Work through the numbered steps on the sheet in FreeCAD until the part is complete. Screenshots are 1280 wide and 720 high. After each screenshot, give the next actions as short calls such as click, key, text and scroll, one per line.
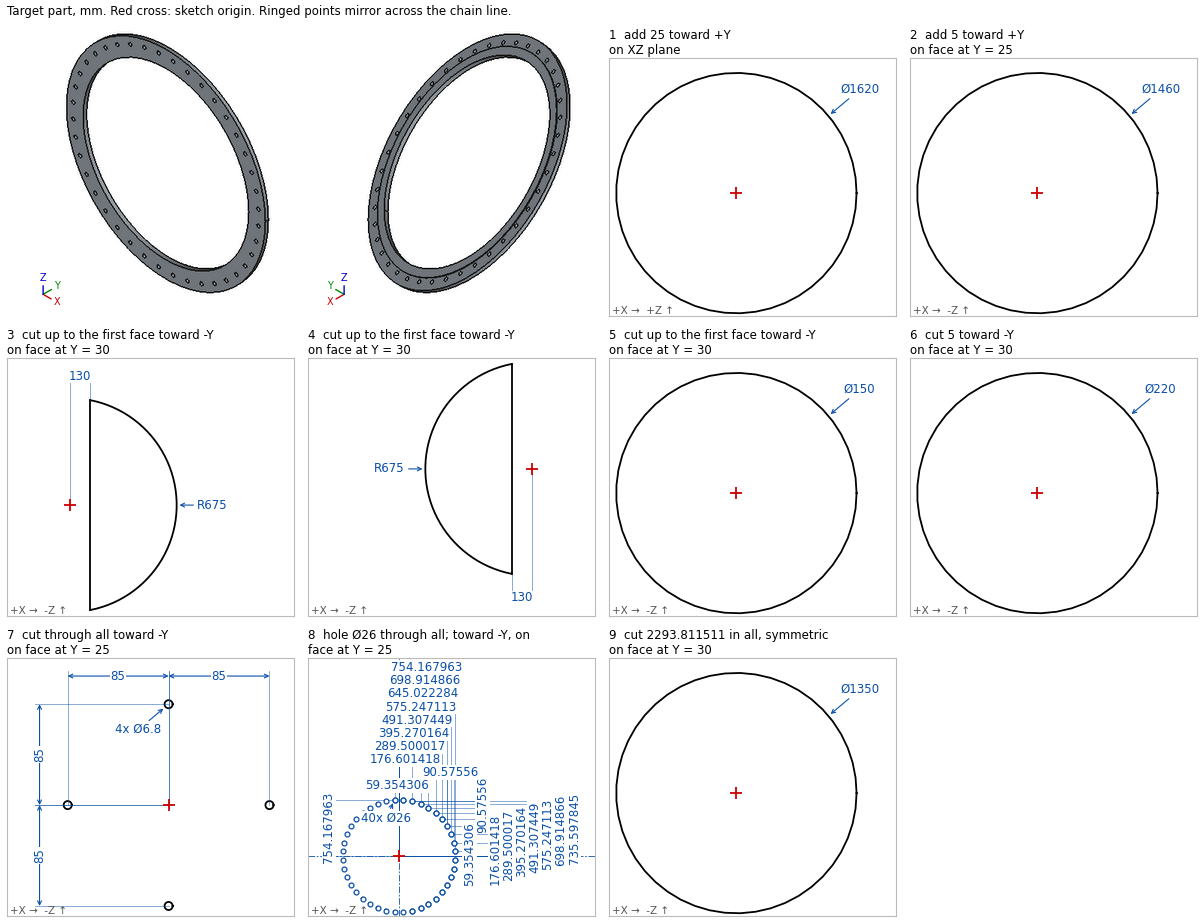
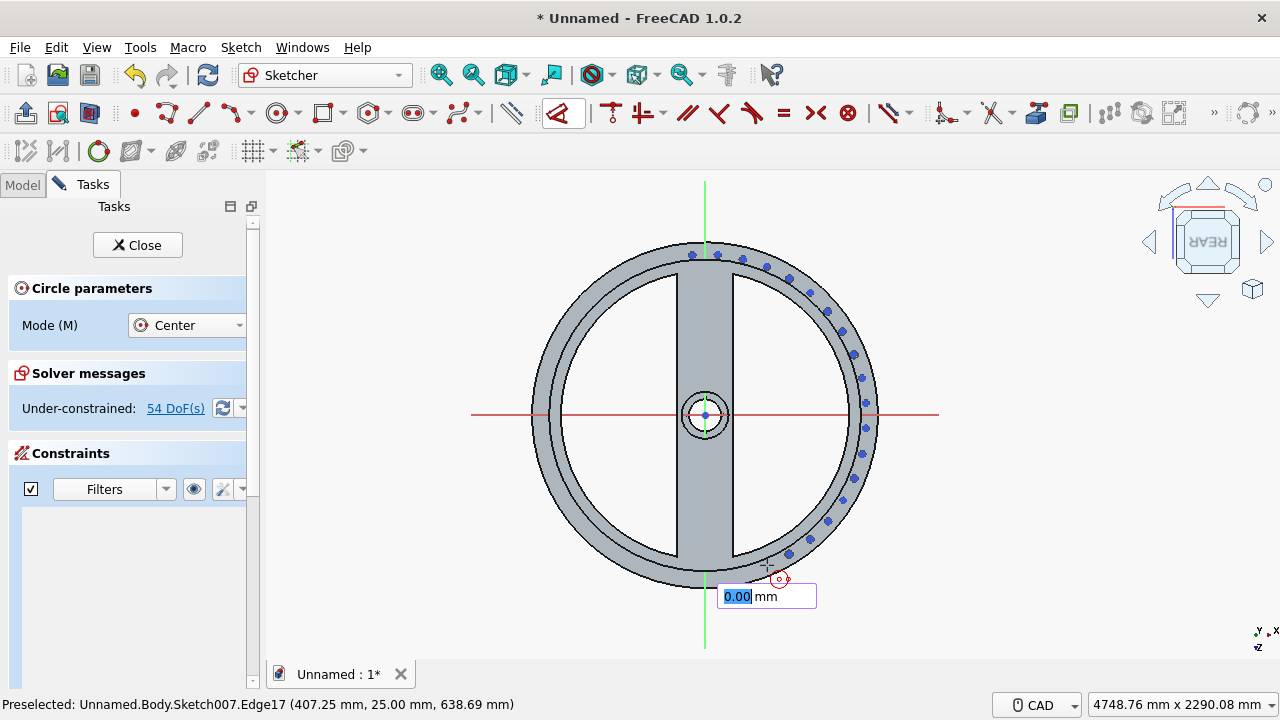
scroll(769, 563, up, 9)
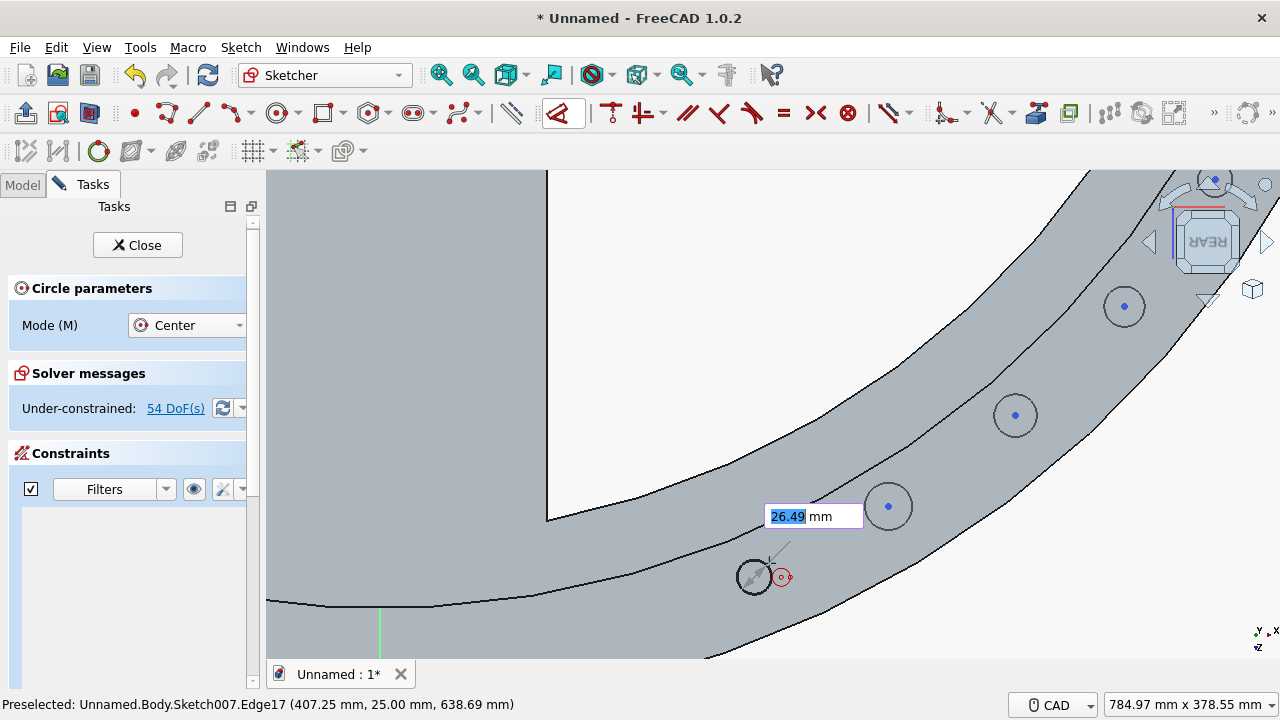
click(765, 556)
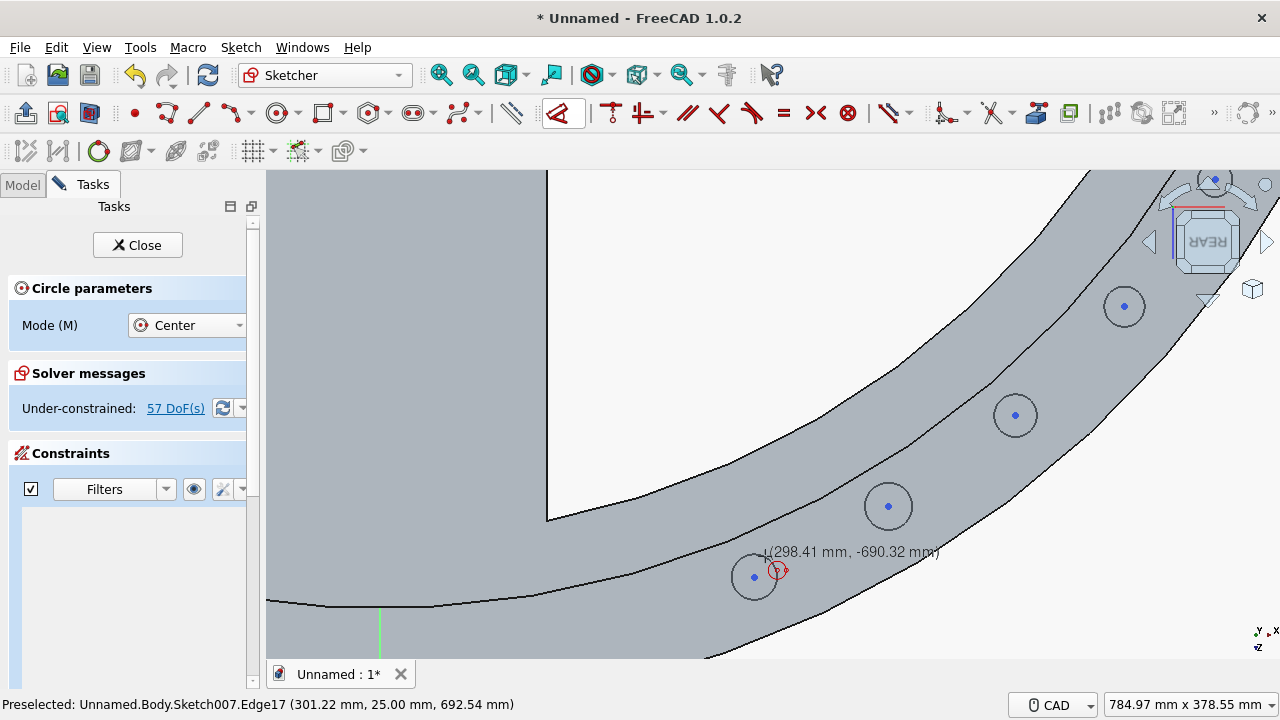
scroll(608, 615, up, 2)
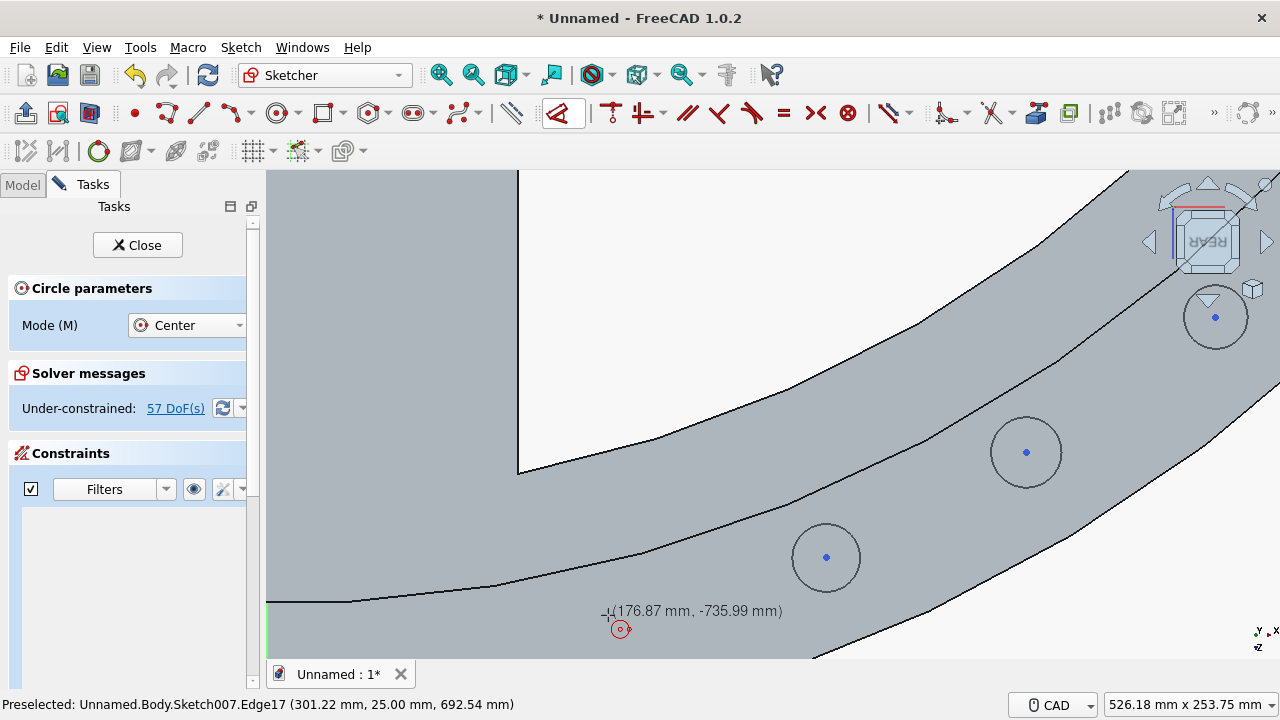
scroll(759, 566, down, 11)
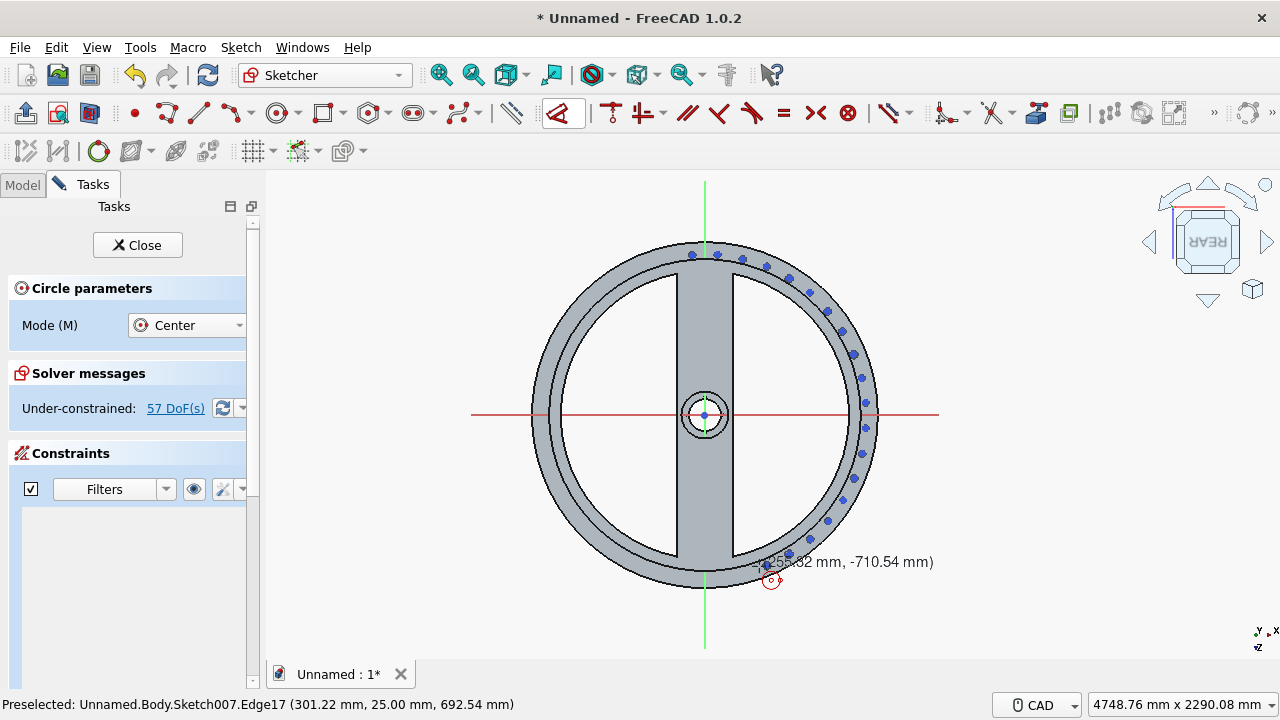
click(743, 572)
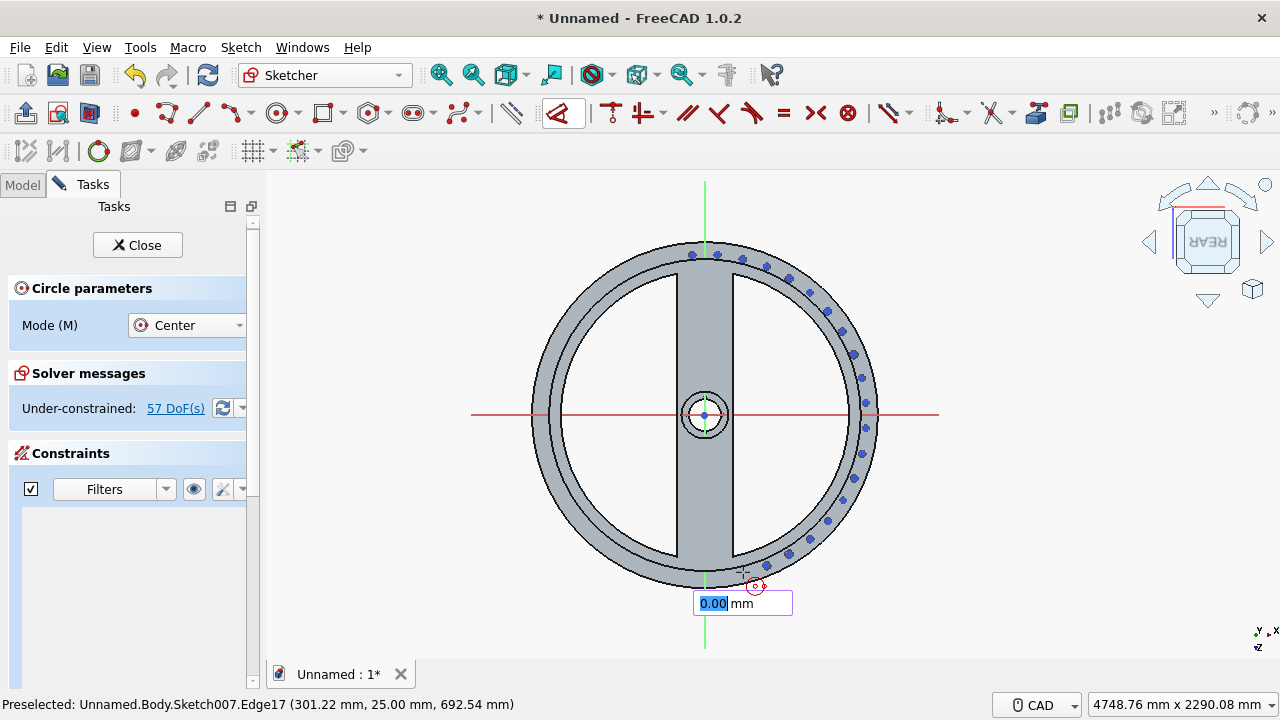
scroll(745, 570, up, 9)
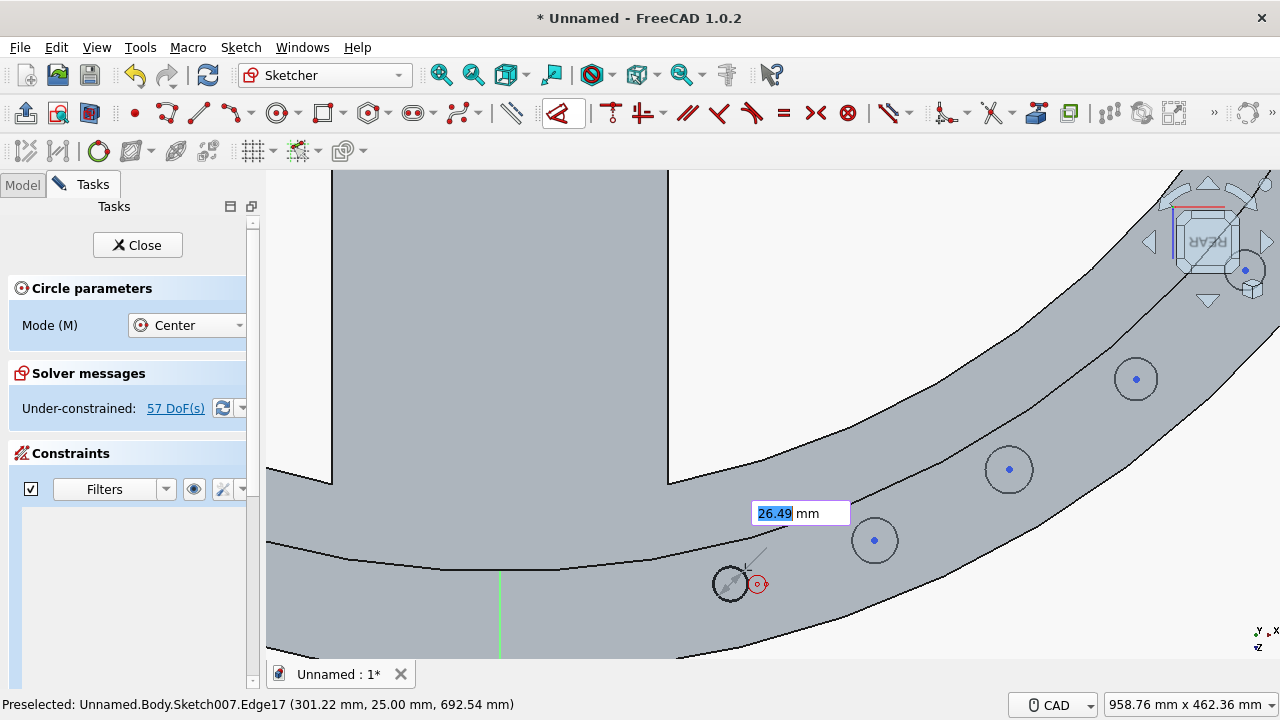
click(740, 567)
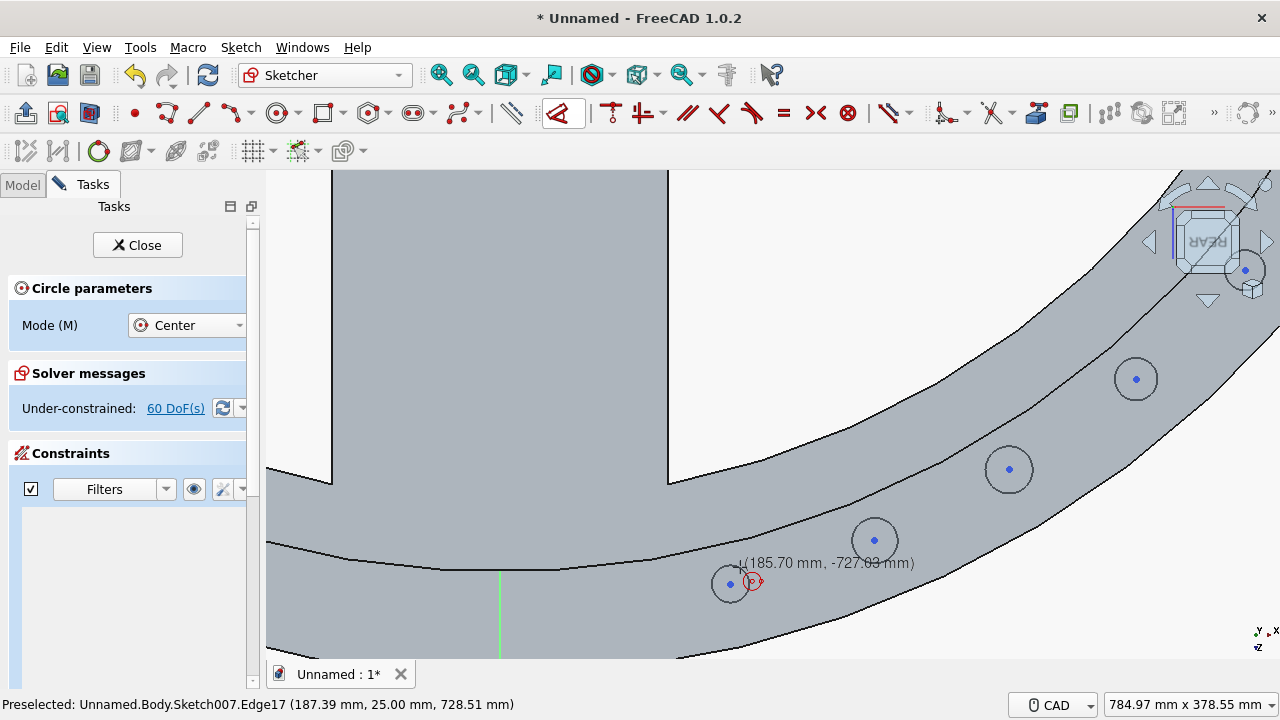
scroll(577, 603, up, 2)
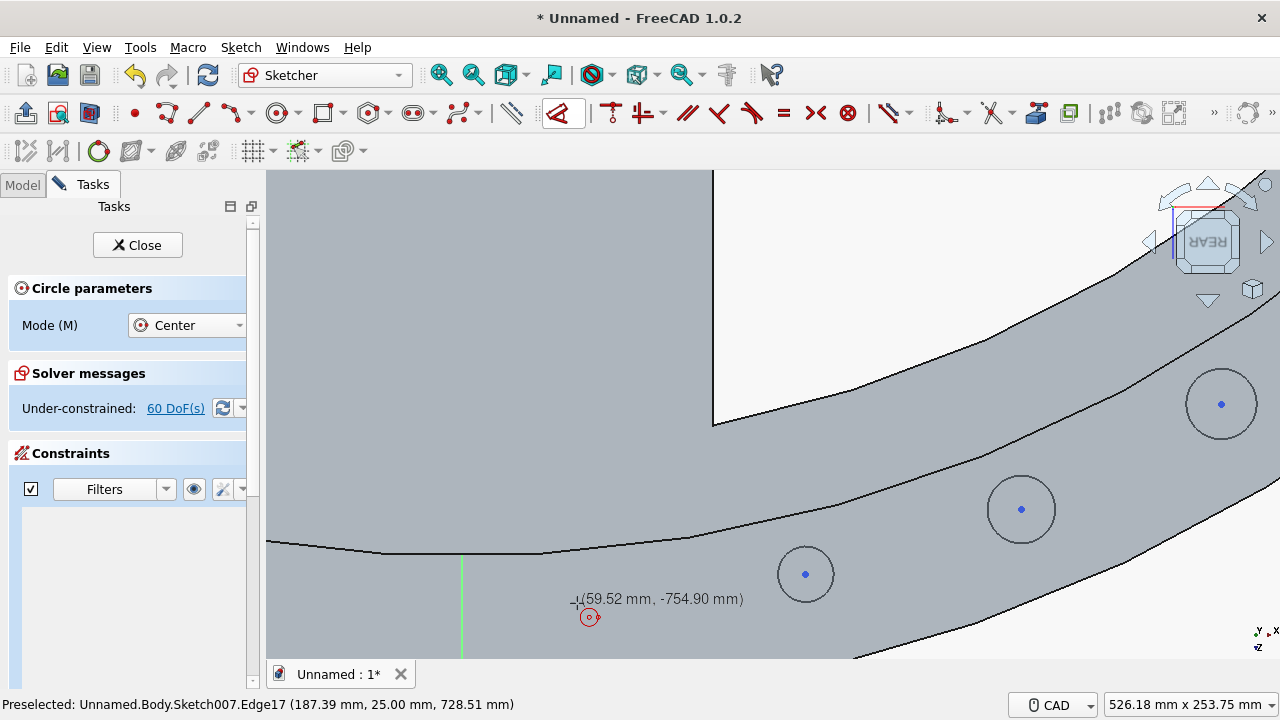
scroll(735, 572, down, 11)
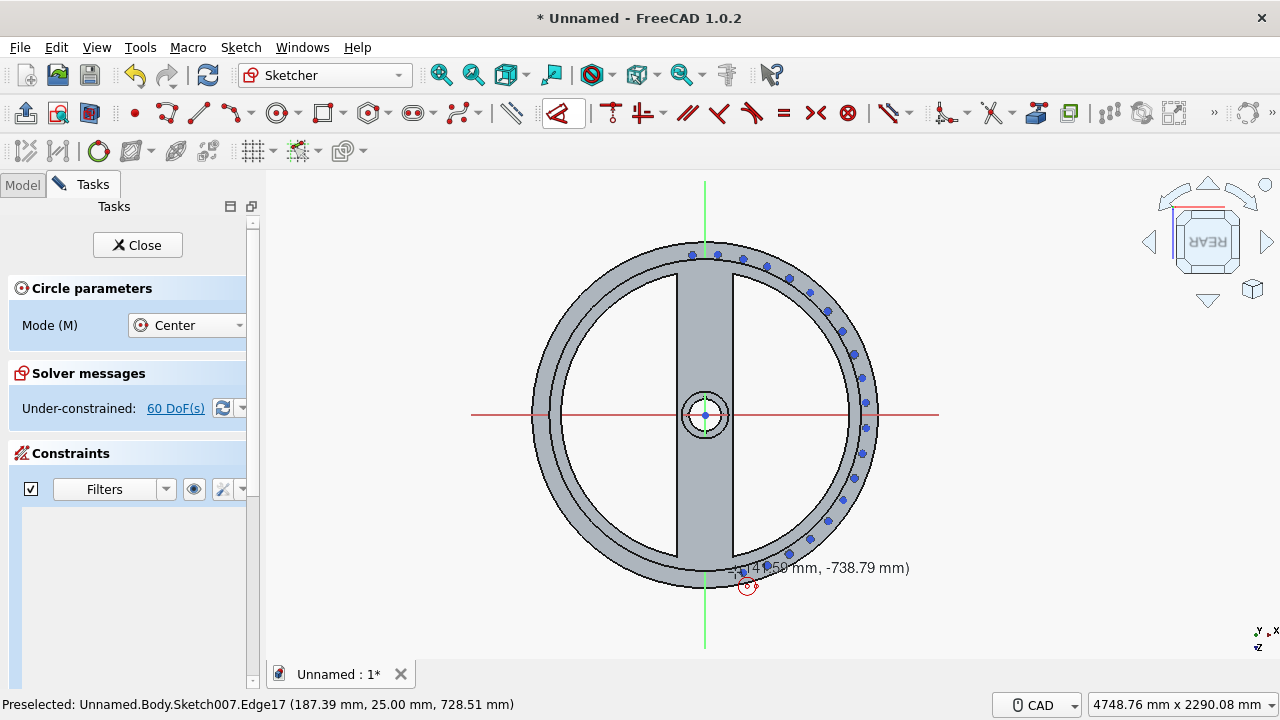
scroll(718, 576, up, 2)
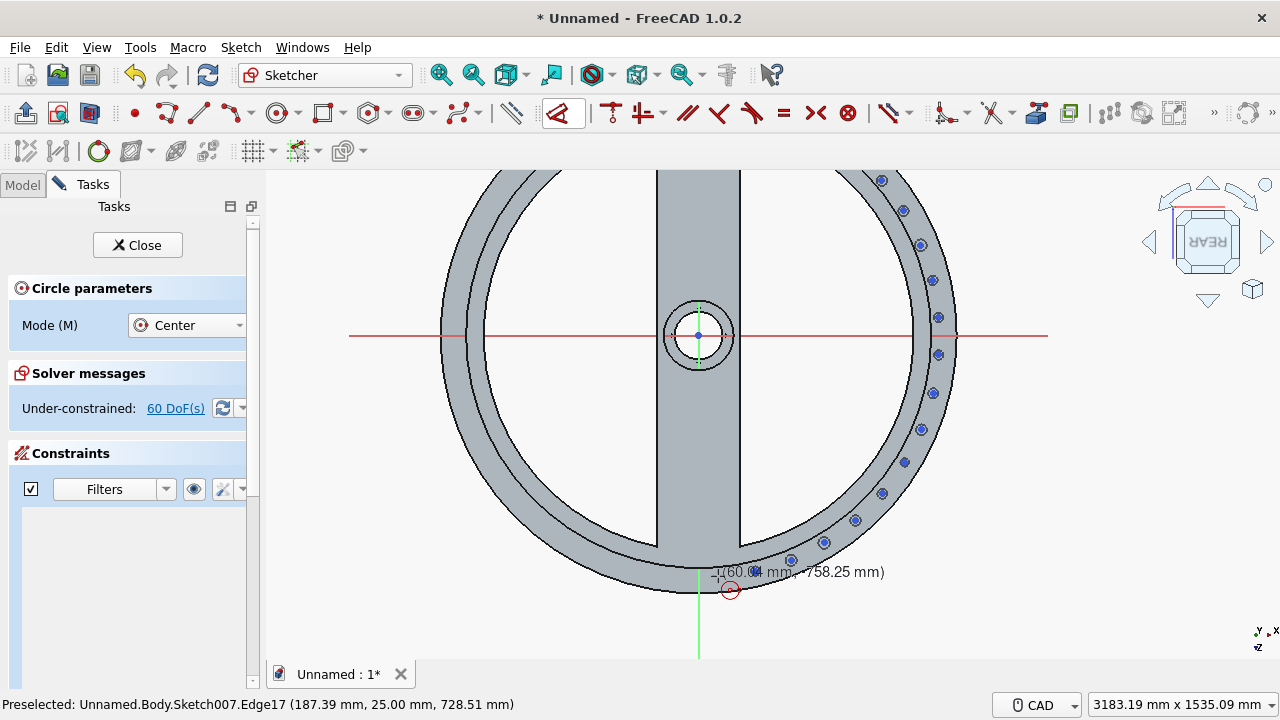
click(718, 576)